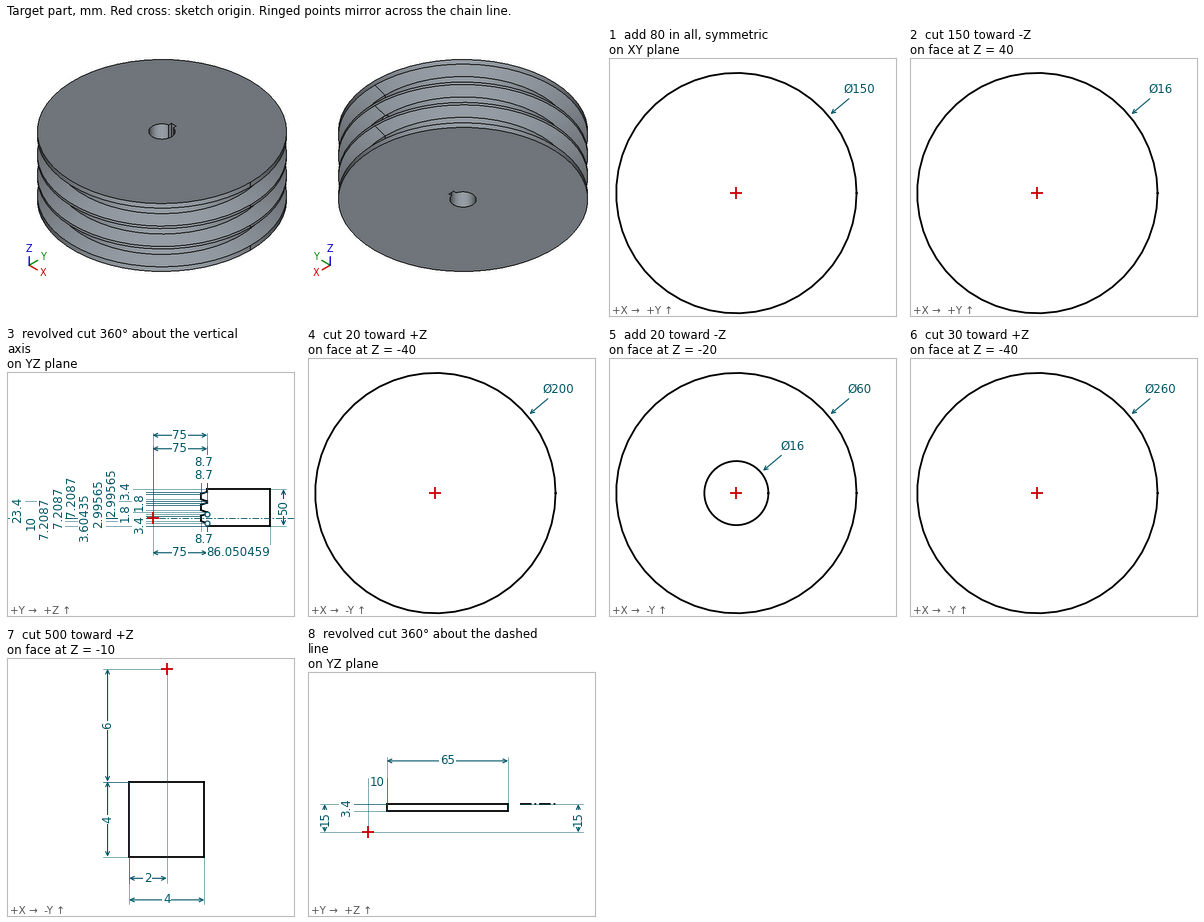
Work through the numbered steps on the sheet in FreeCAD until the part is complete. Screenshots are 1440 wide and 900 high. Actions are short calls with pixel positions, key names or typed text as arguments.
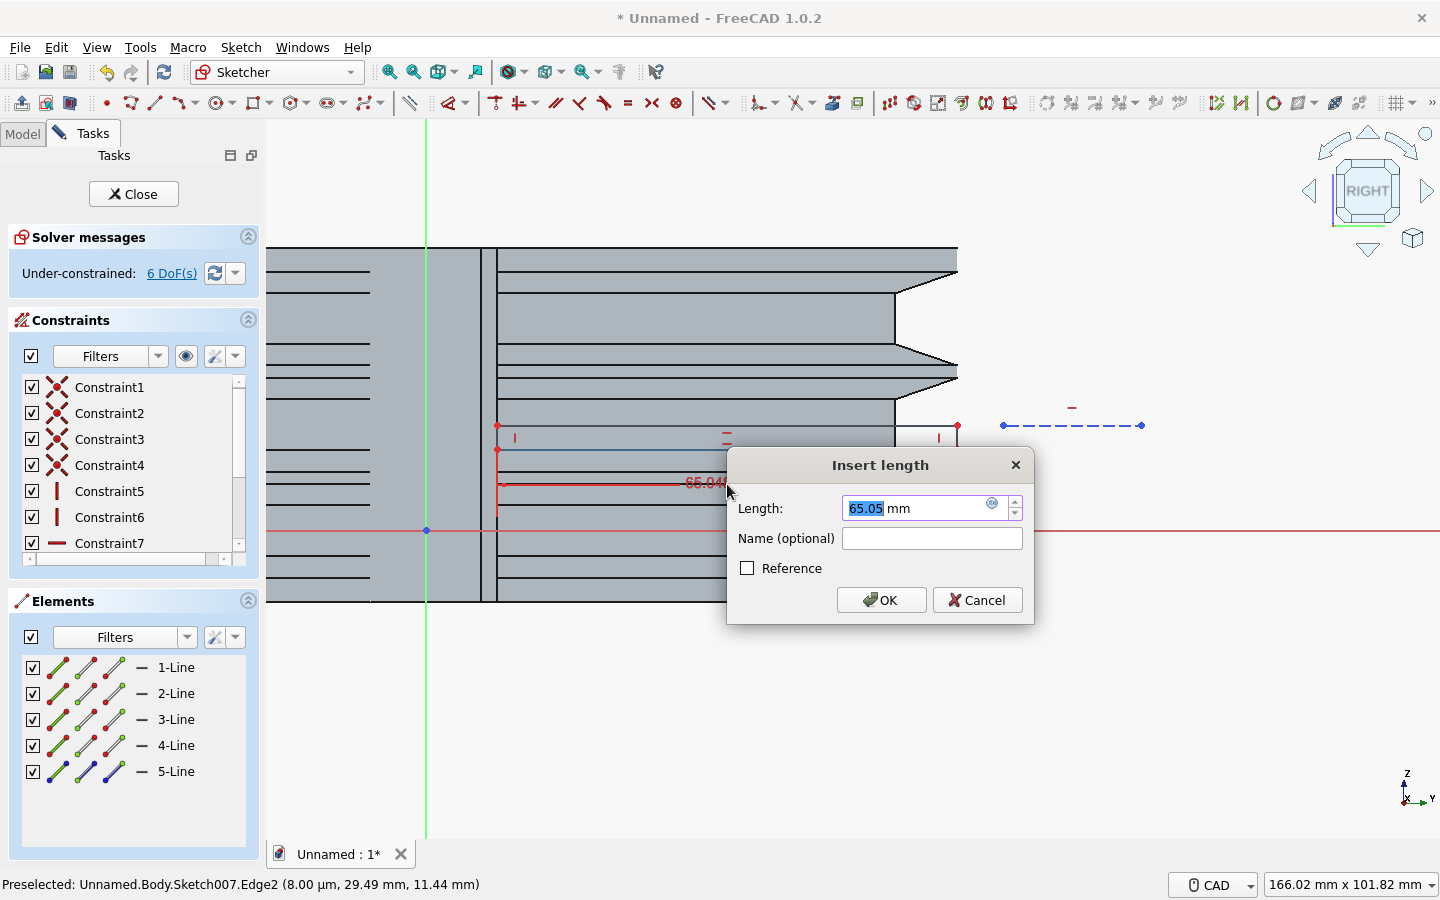
text(65)
key(Return)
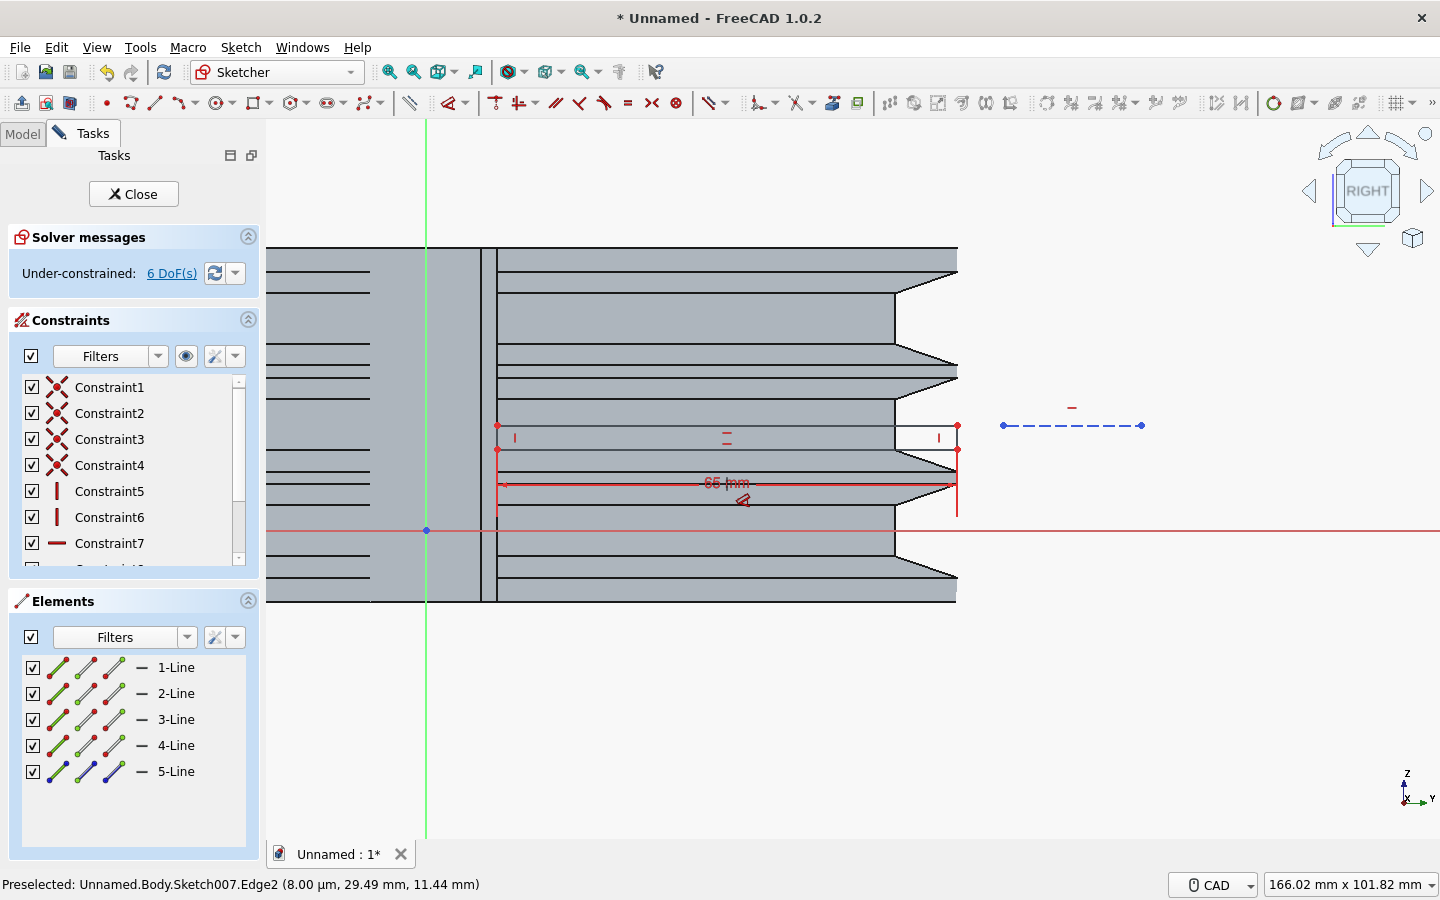
scroll(497, 436, up, 3)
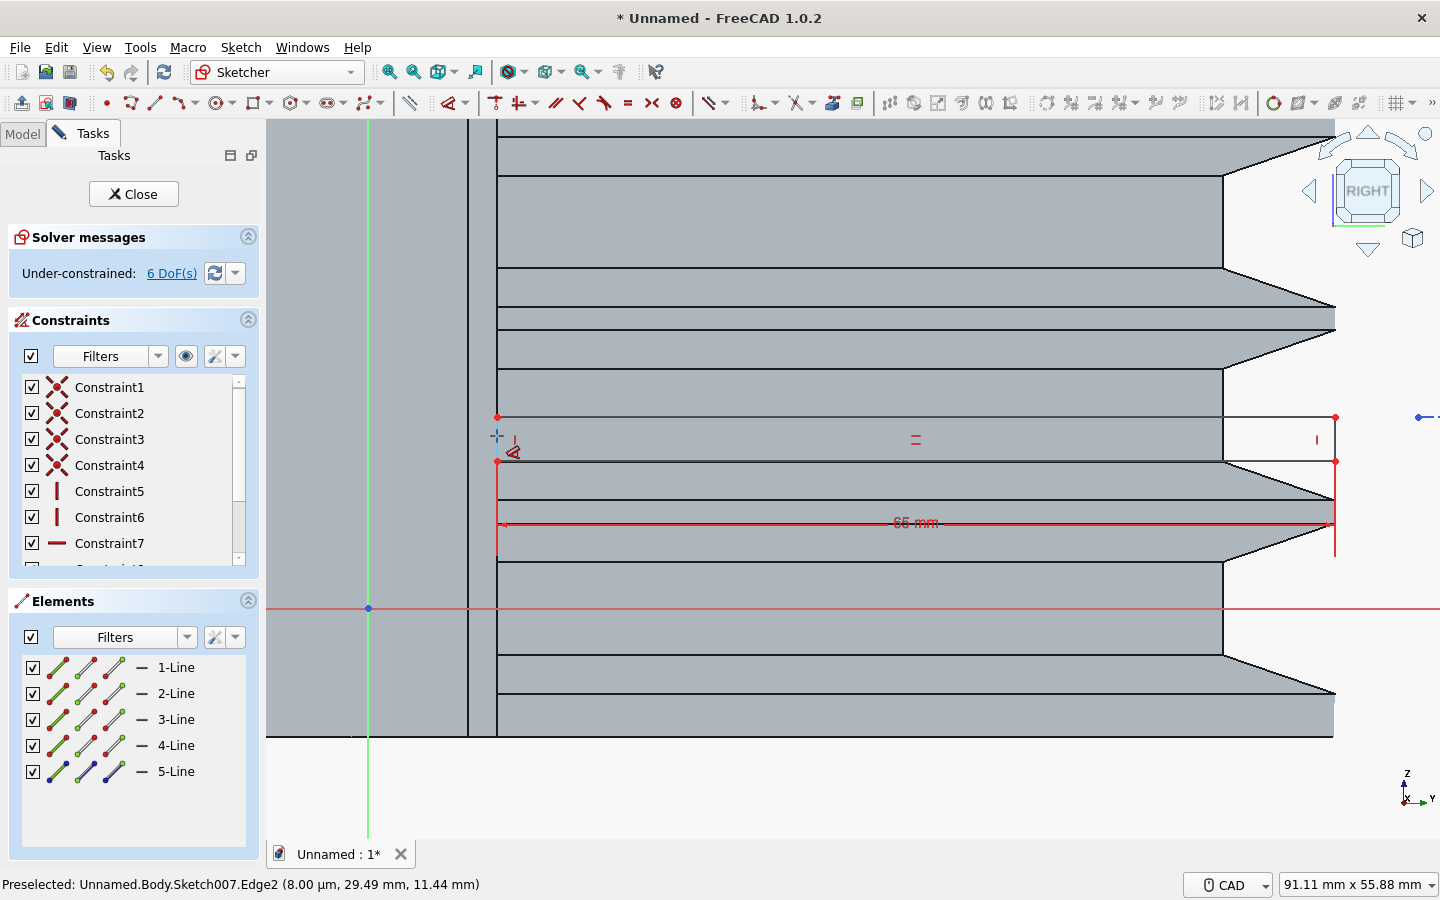
click(497, 435)
click(463, 439)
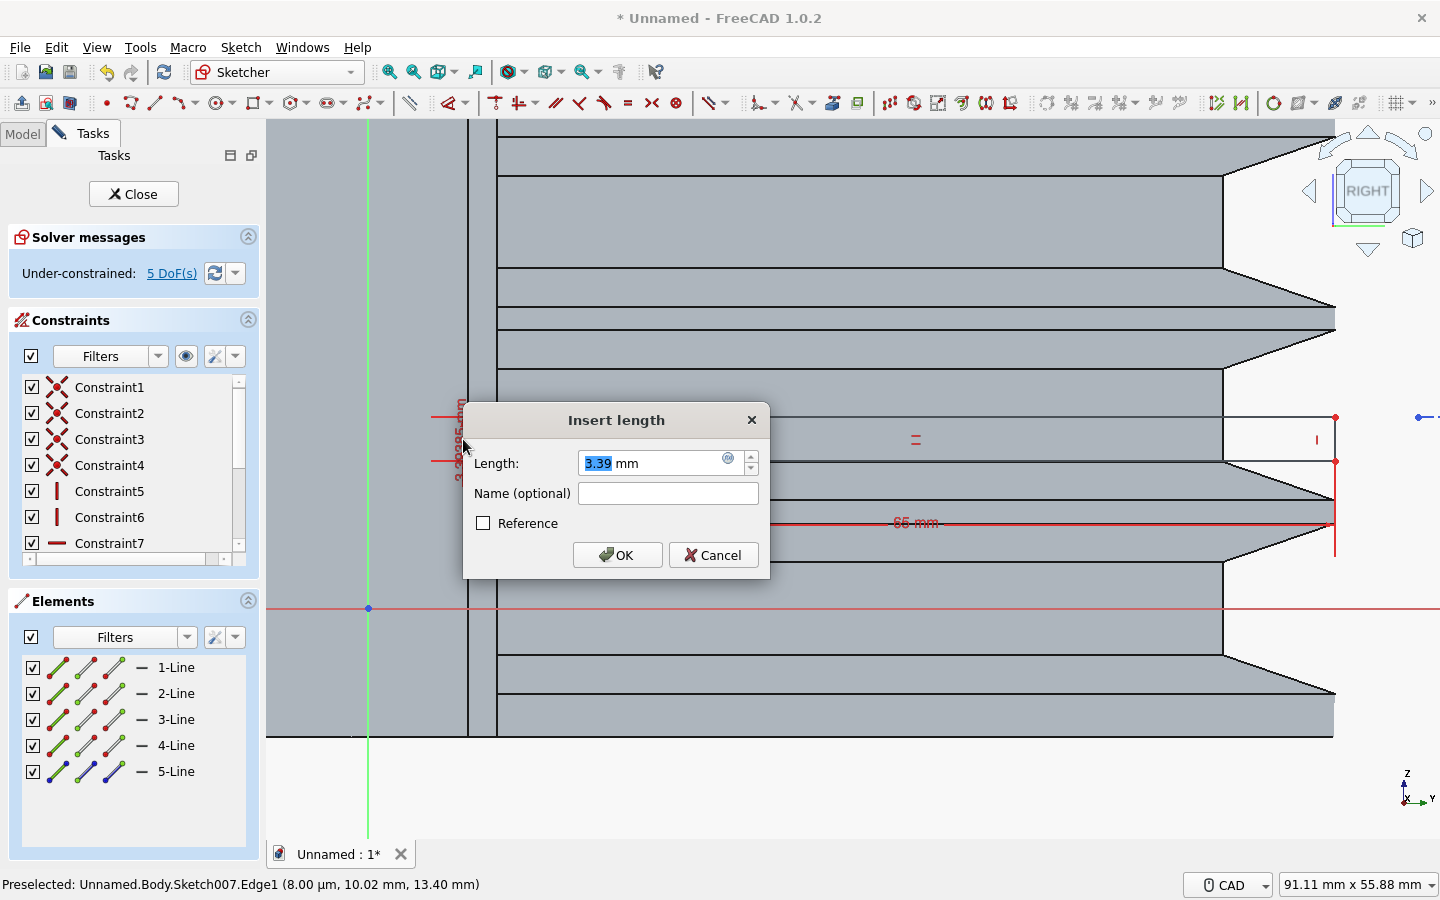
text(3.4)
key(Return)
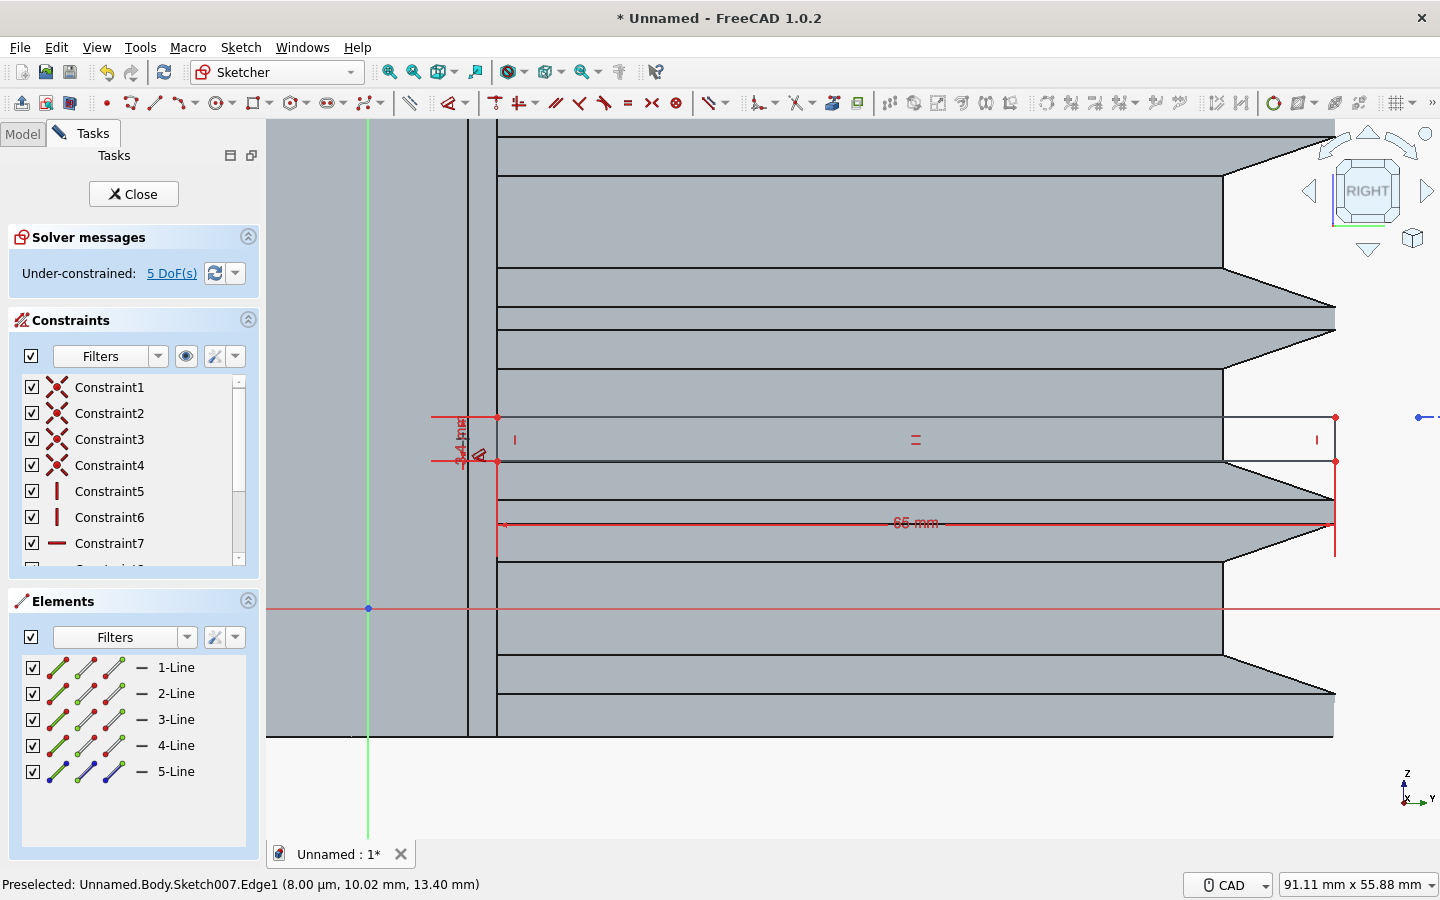
click(497, 417)
click(433, 643)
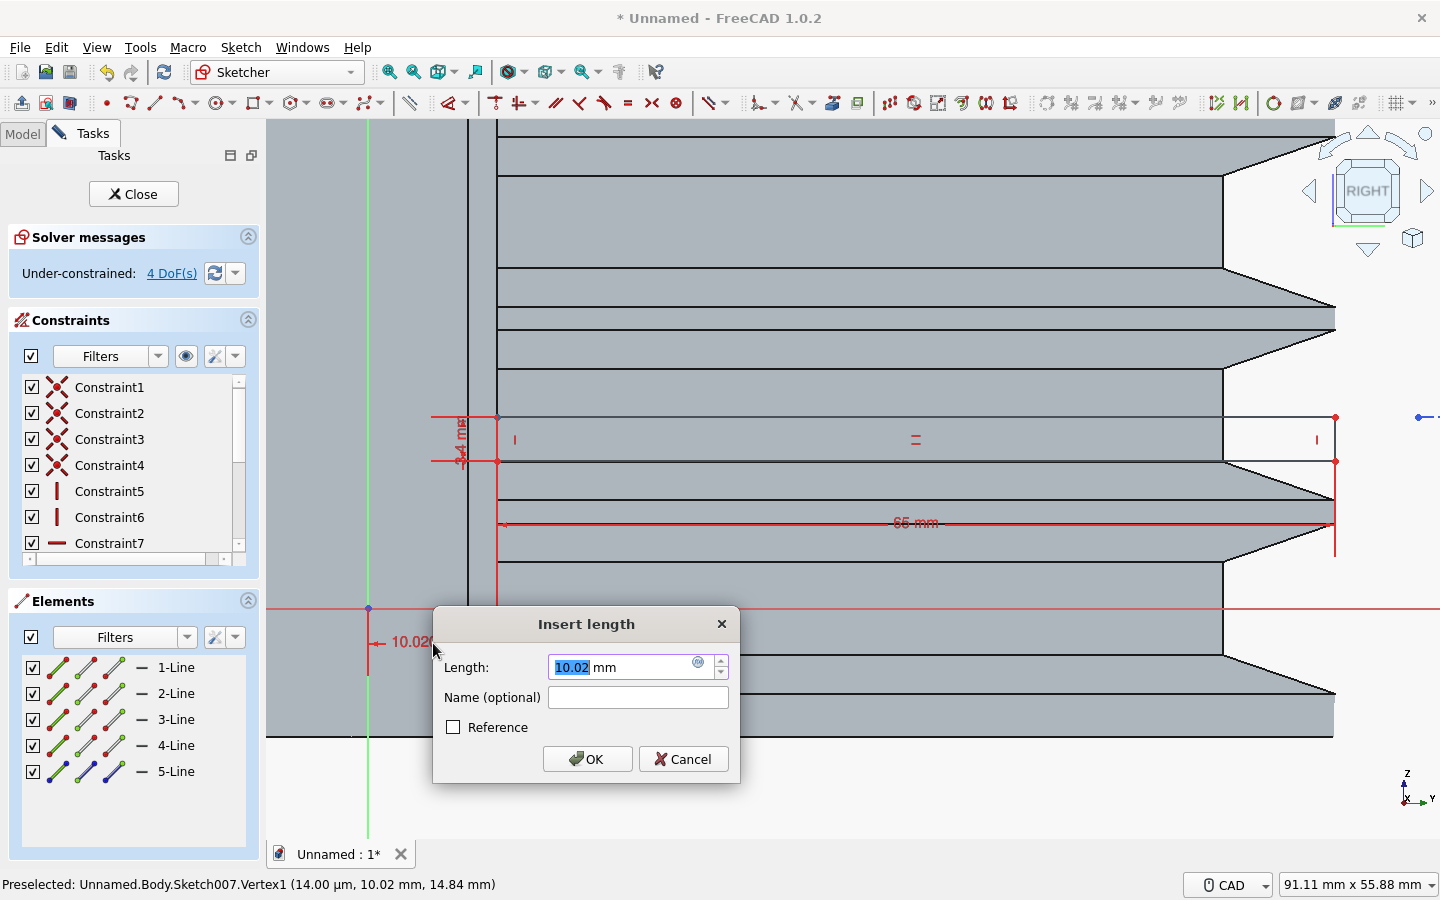
text(10)
key(Return)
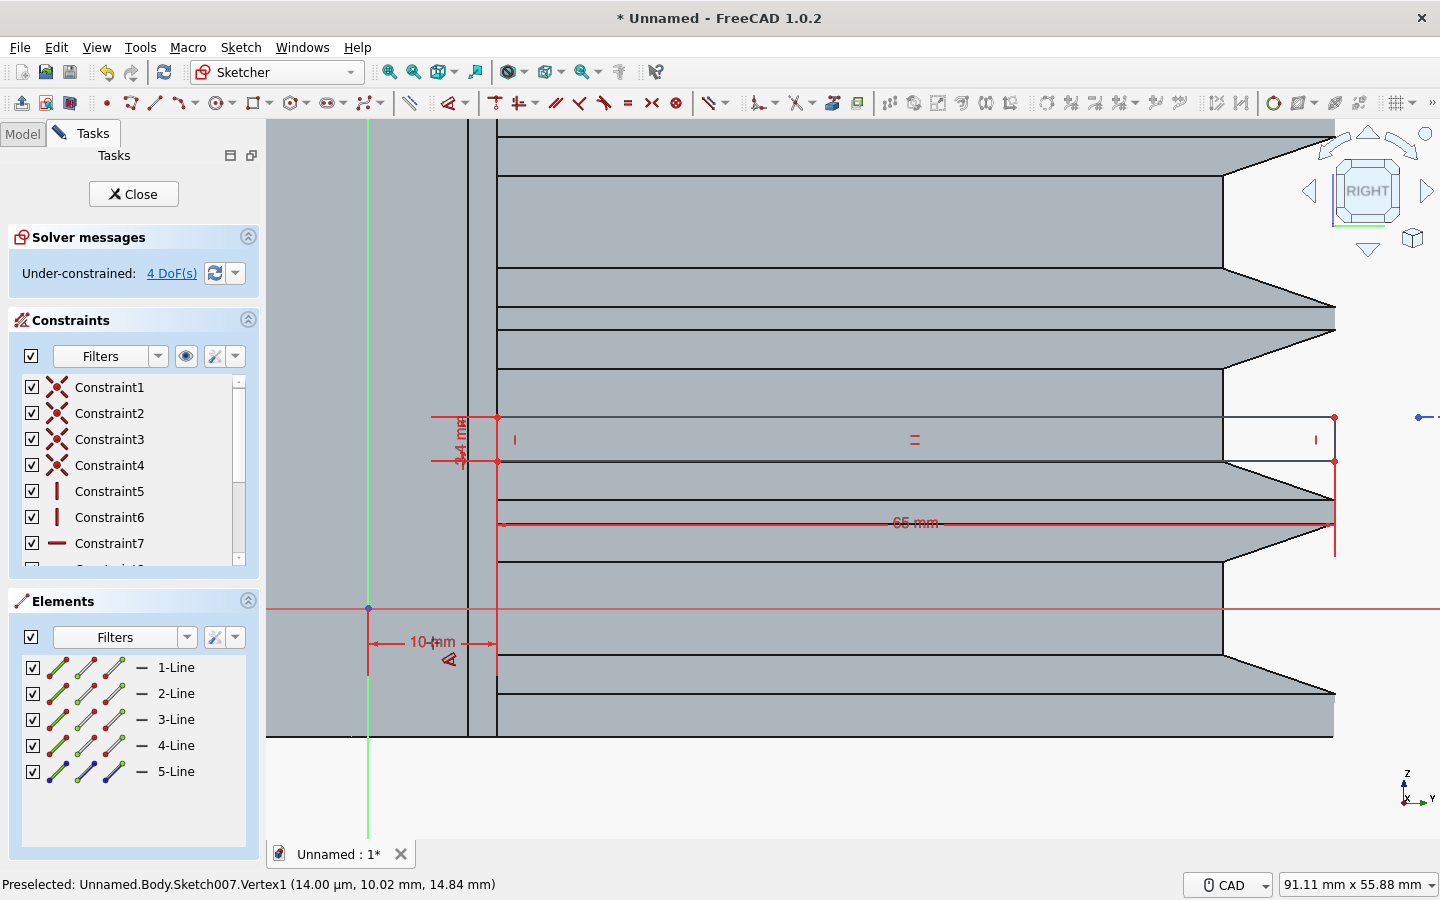
click(497, 417)
click(334, 513)